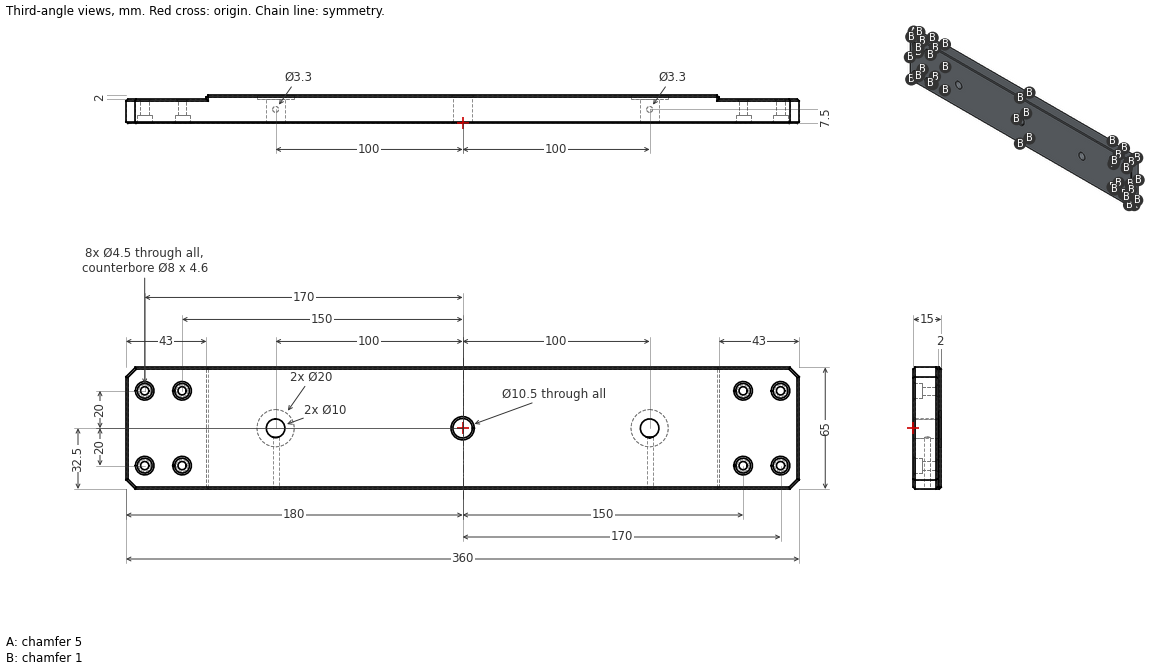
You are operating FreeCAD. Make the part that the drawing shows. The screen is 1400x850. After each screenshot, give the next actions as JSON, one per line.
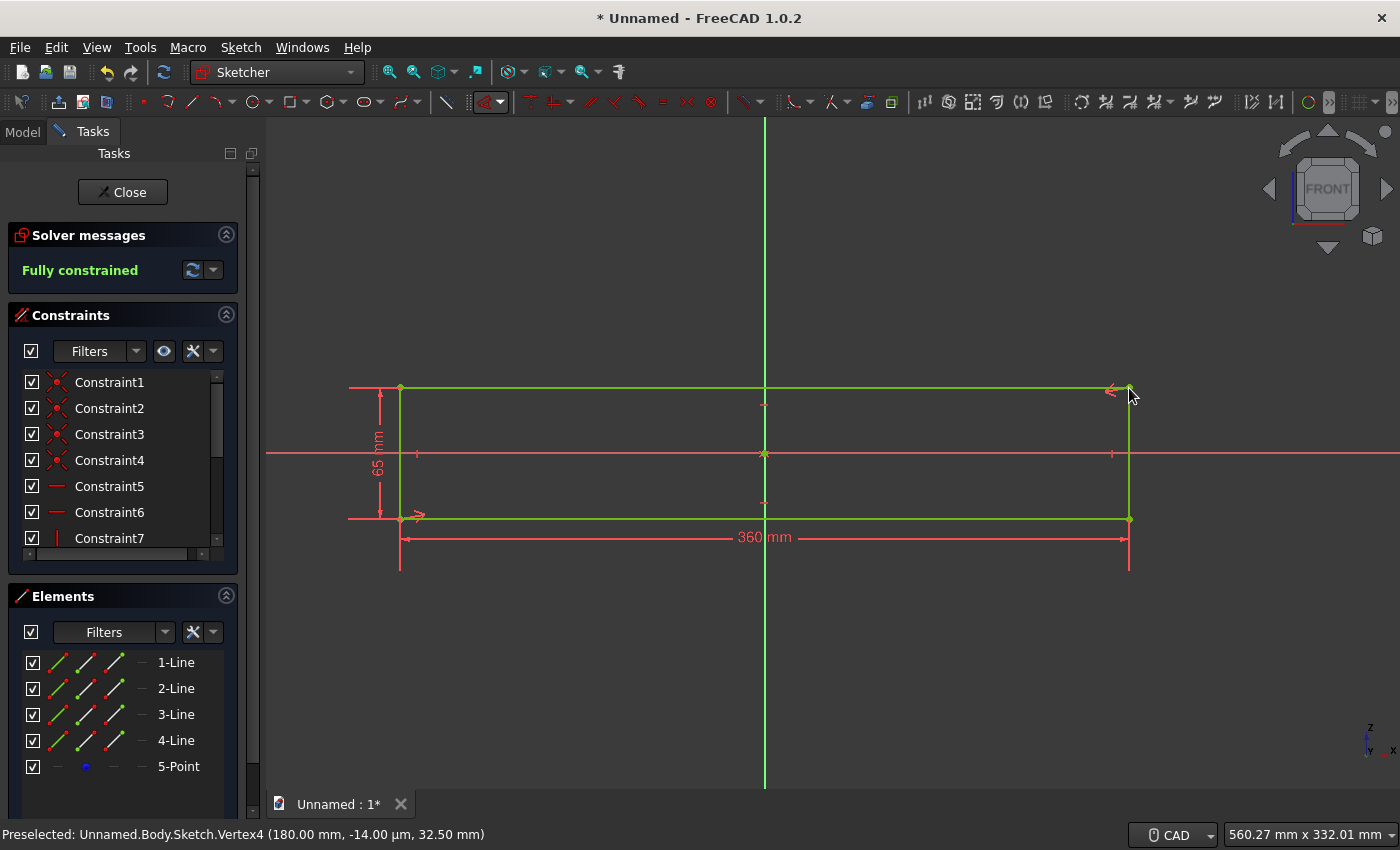
{"action": "left_click", "coordinate": [123, 192]}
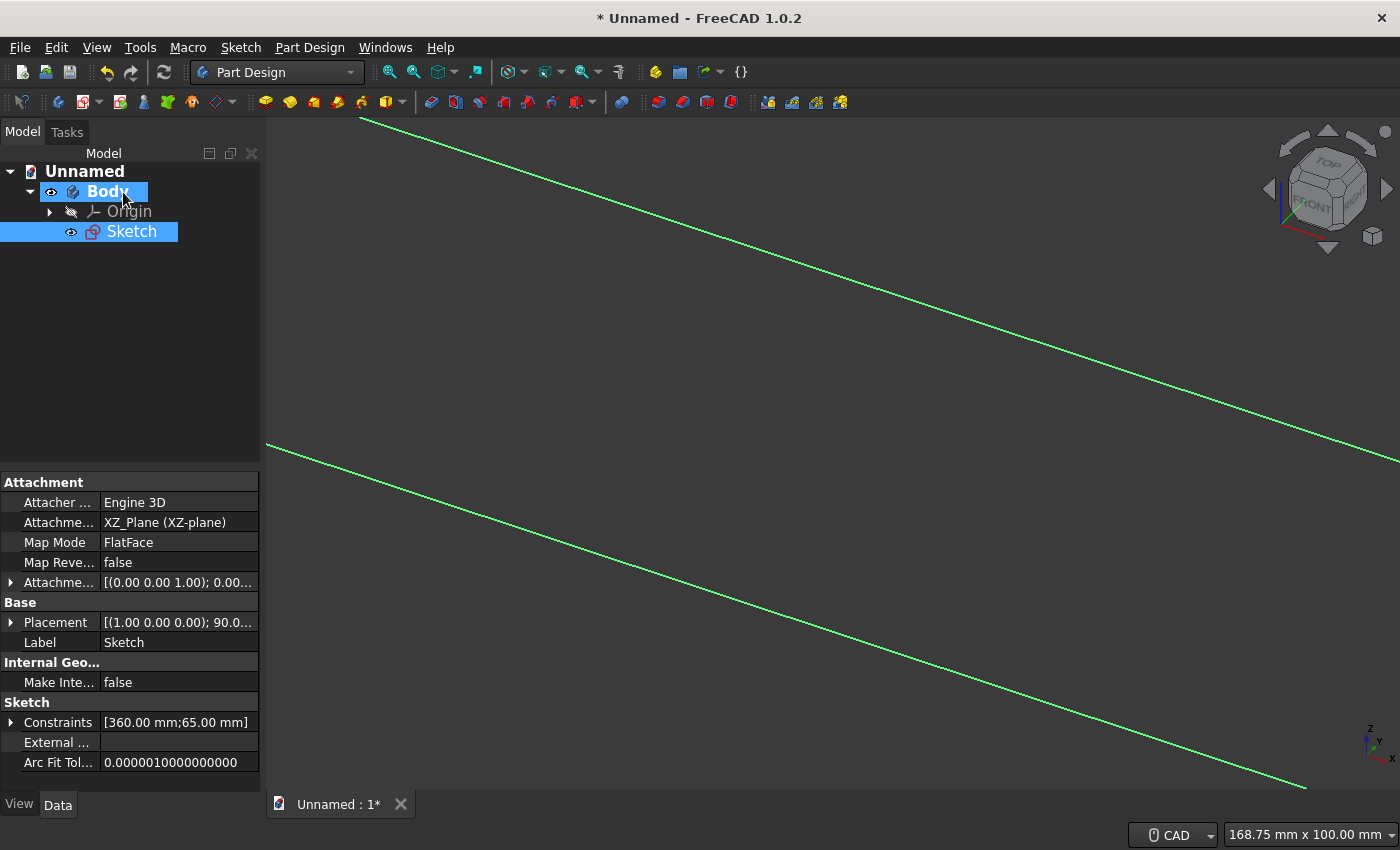
{"action": "left_click", "coordinate": [266, 102]}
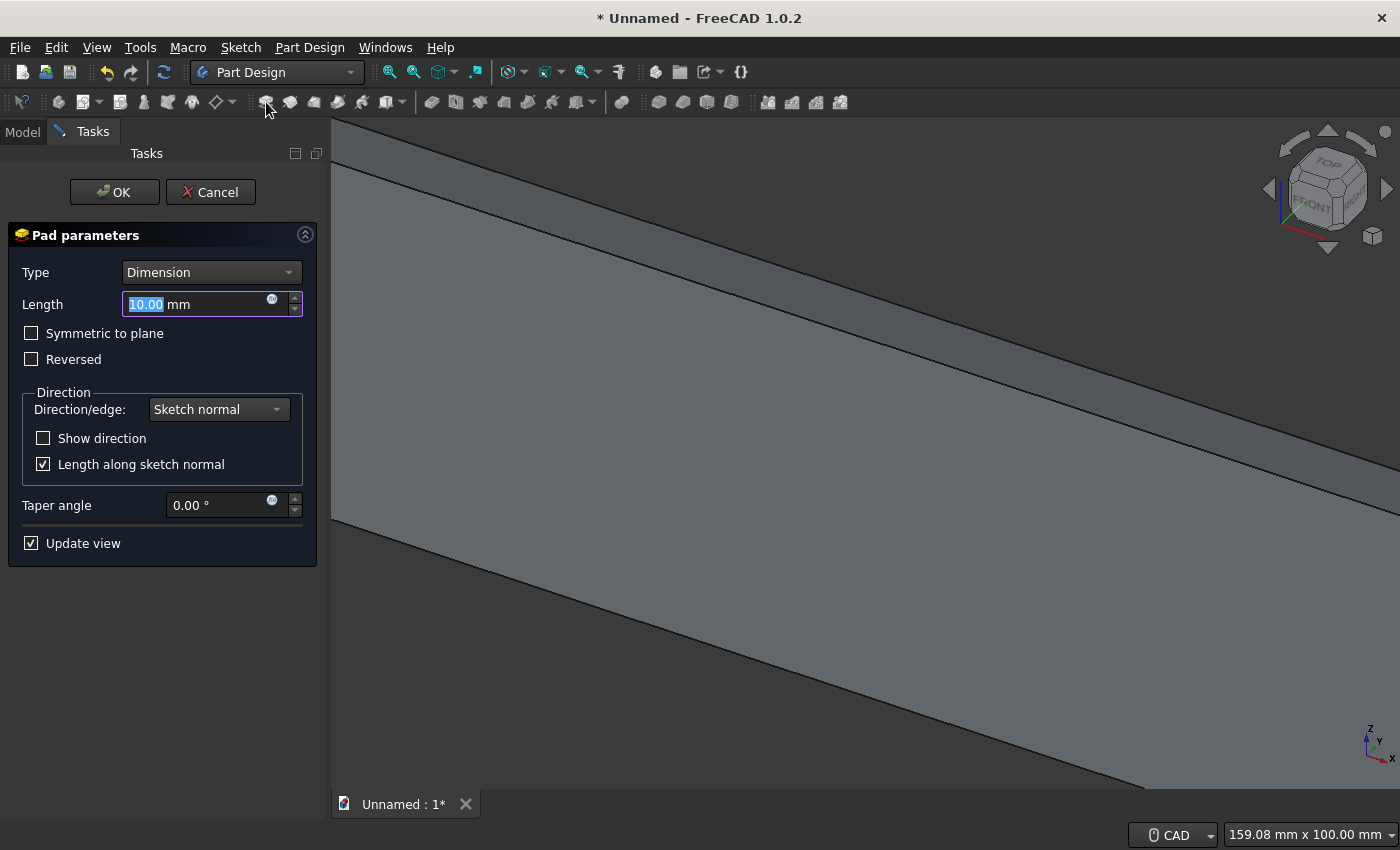
{"action": "type", "text": "15"}
{"action": "key", "text": "Tab"}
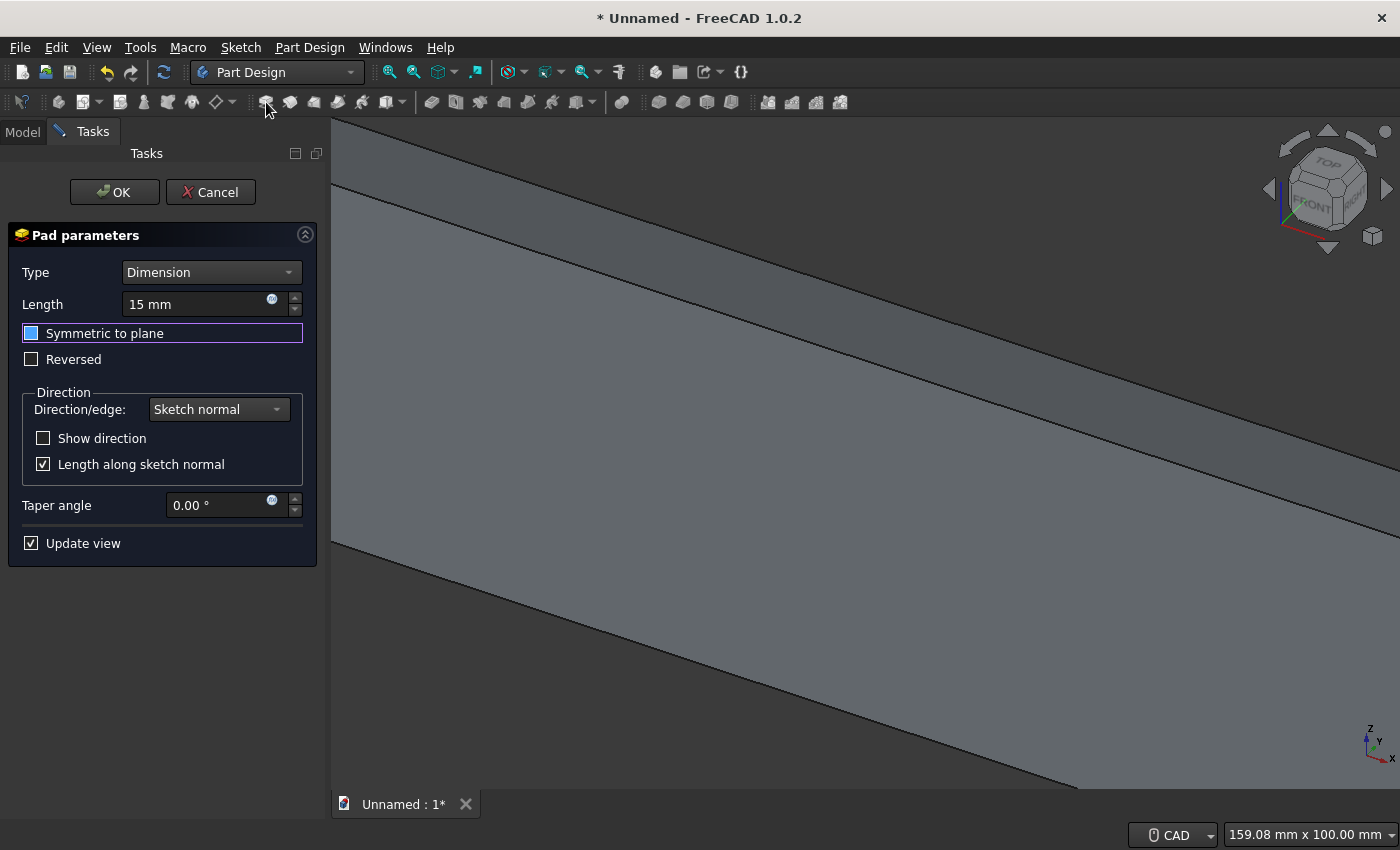
{"action": "left_click", "coordinate": [30, 359]}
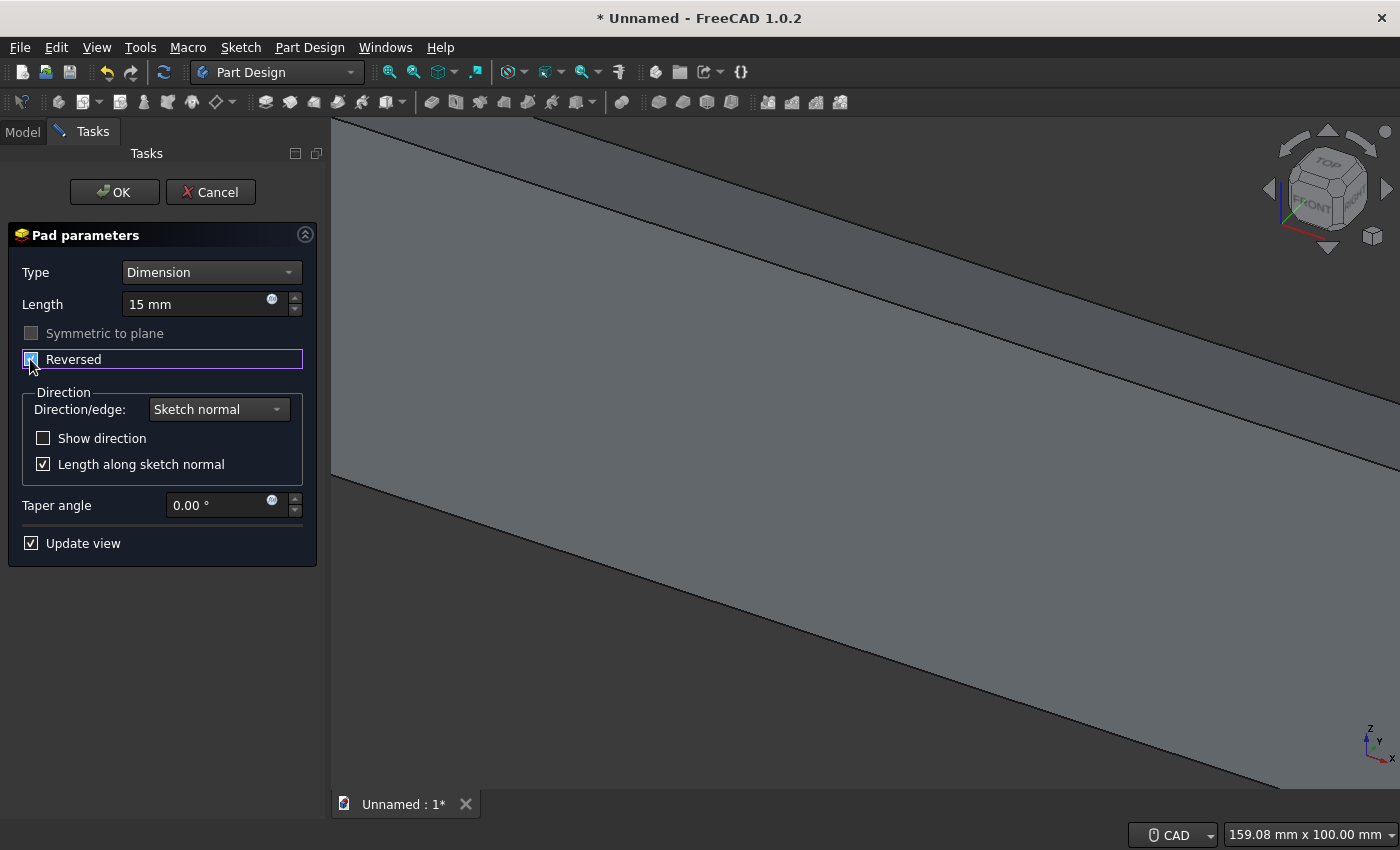
{"action": "left_click", "coordinate": [115, 192]}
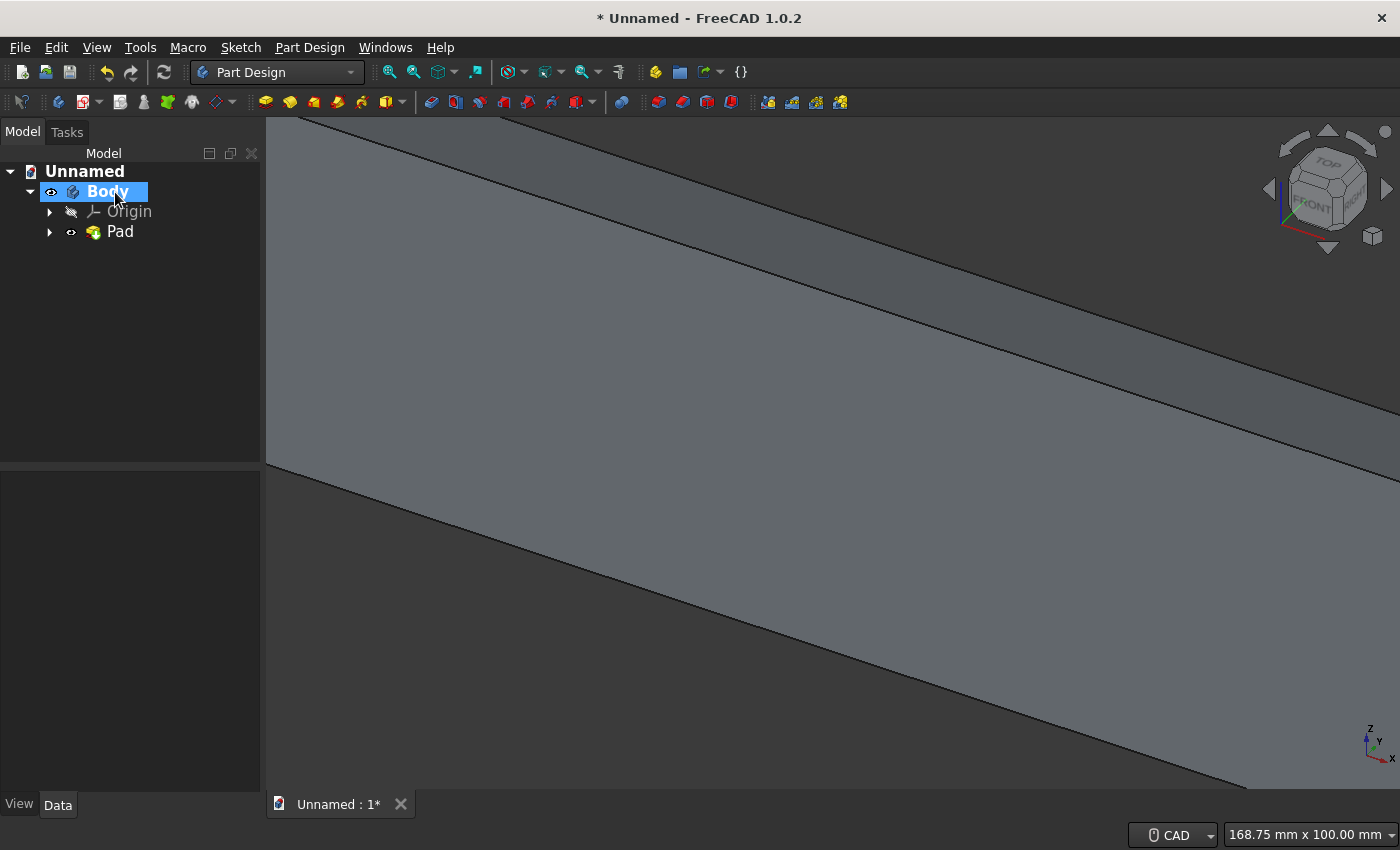
{"action": "left_click", "coordinate": [390, 72]}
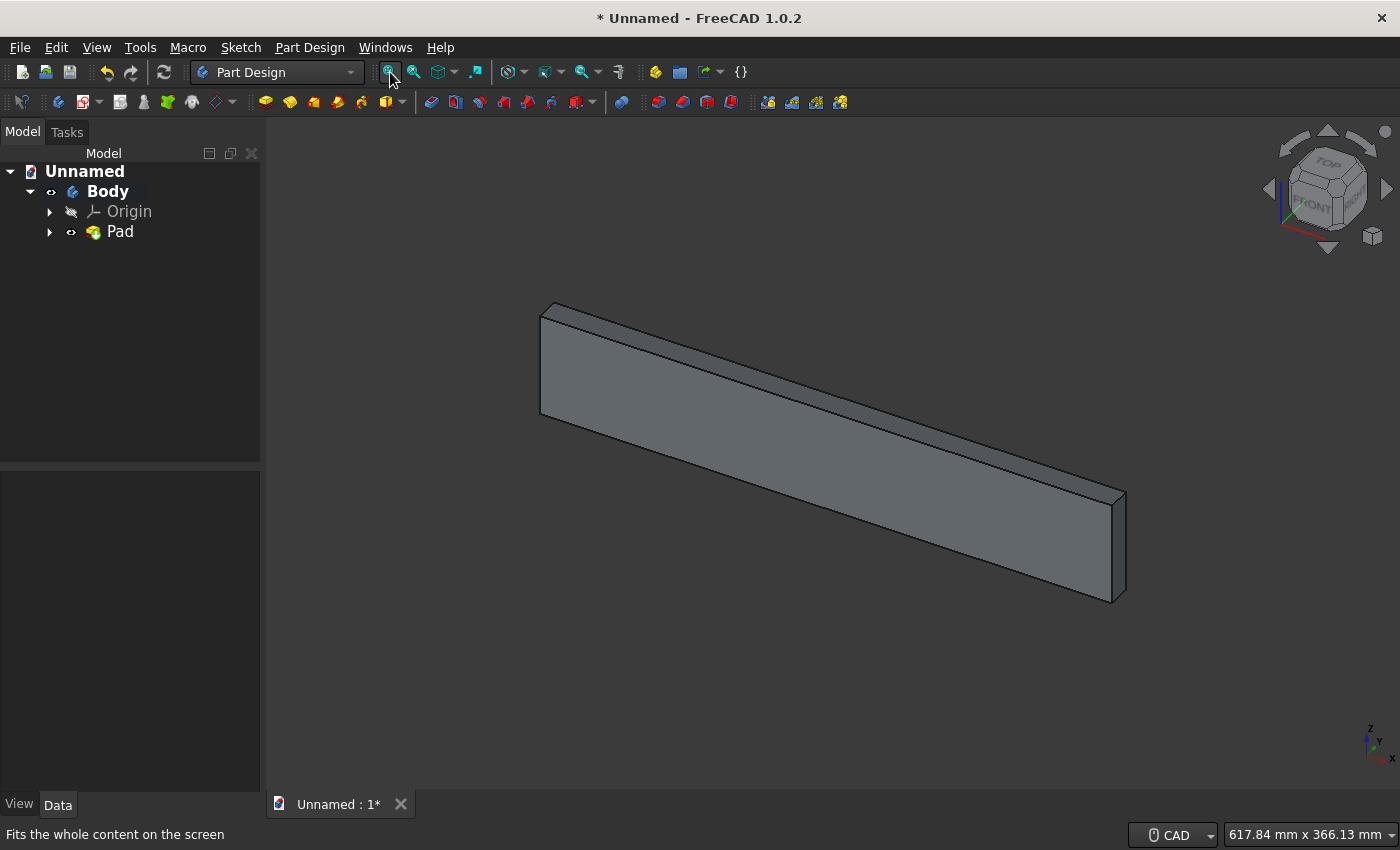
{"action": "key", "text": "4"}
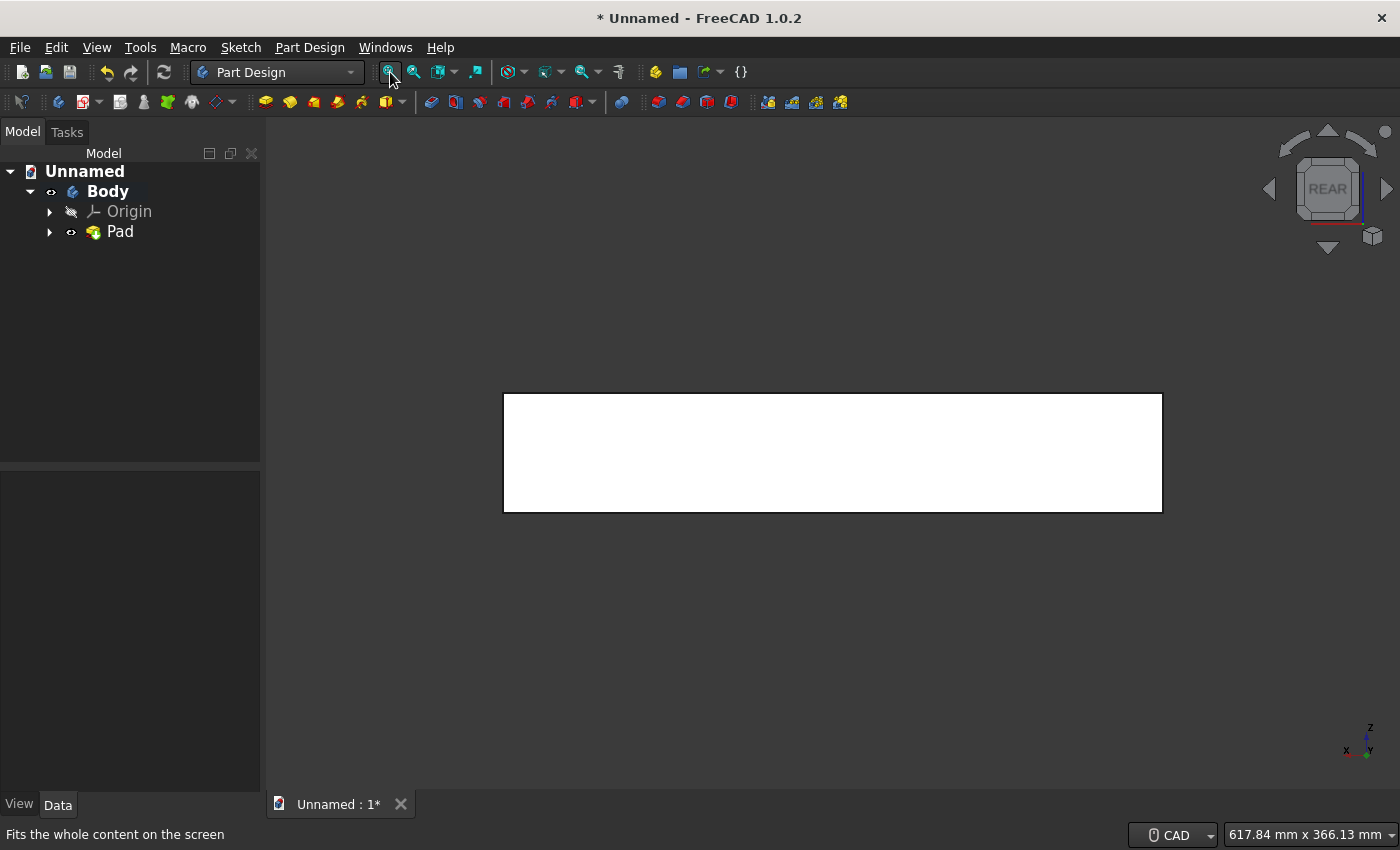
{"action": "left_click", "coordinate": [644, 452]}